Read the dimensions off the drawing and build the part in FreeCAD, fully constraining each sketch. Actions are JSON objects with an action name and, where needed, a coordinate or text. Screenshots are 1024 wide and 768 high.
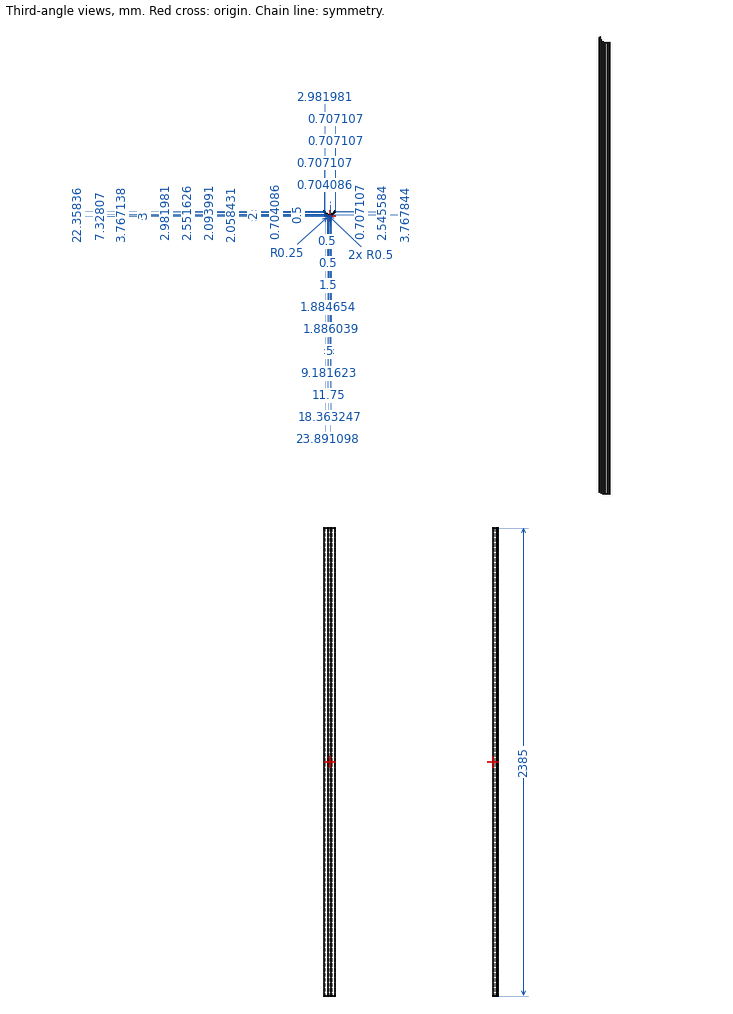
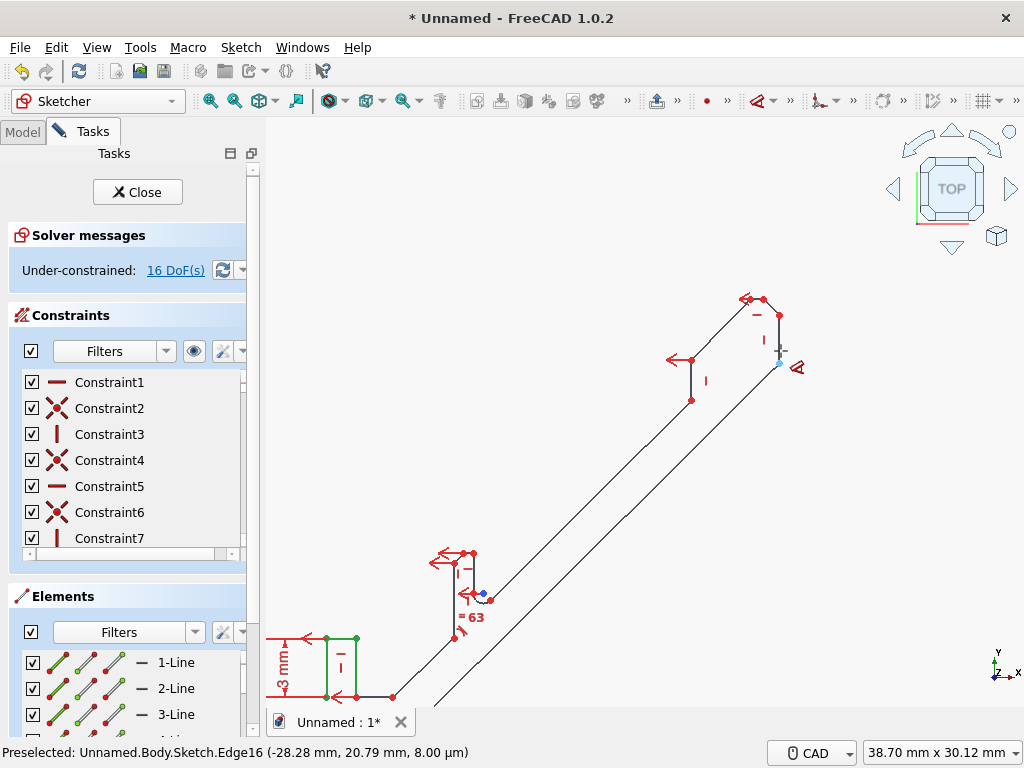
{"action": "left_click", "coordinate": [779, 349]}
{"action": "left_click", "coordinate": [813, 339]}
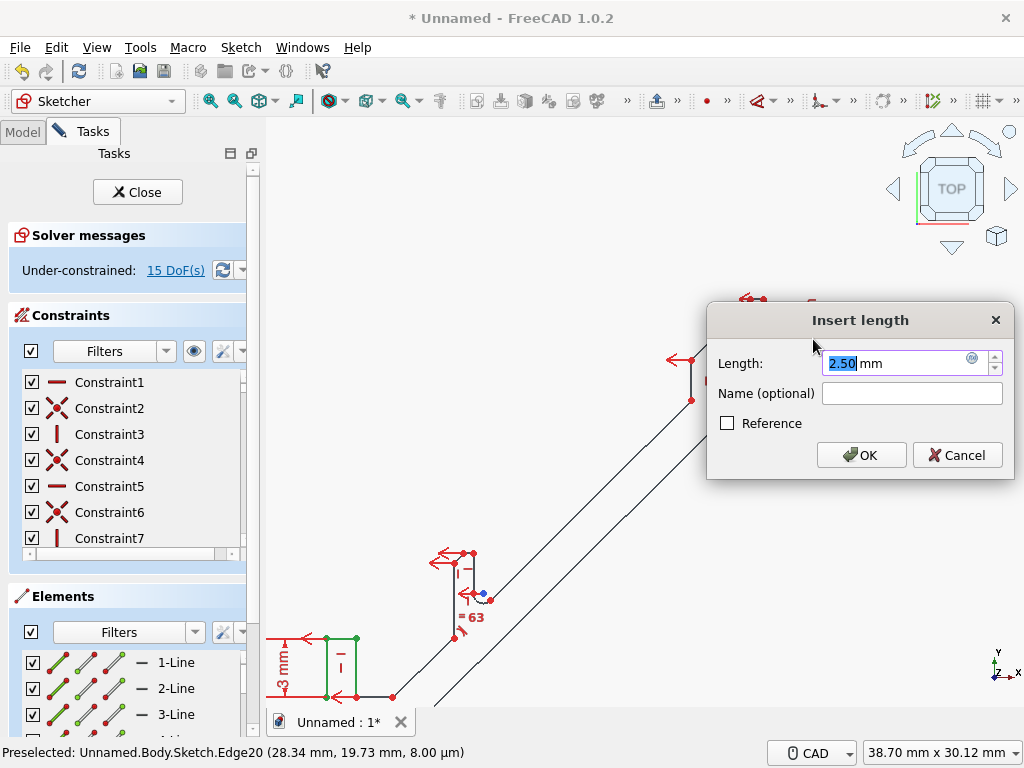
{"action": "type", "text": "2.545584"}
{"action": "key", "text": "Return"}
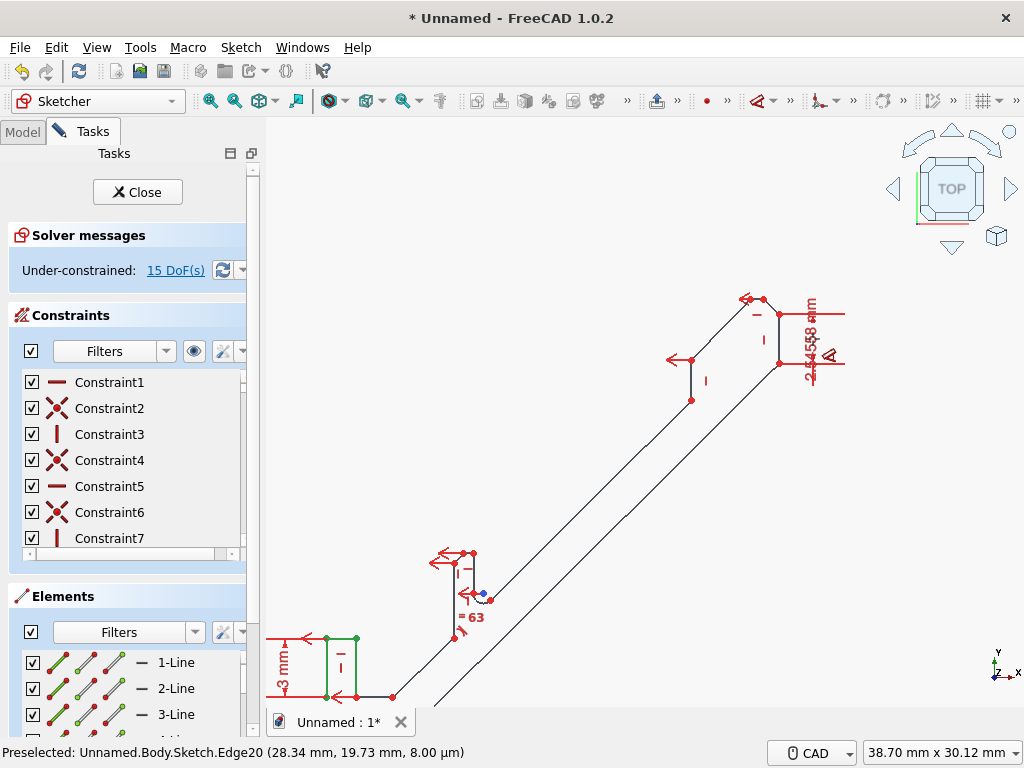
{"action": "scroll", "coordinate": [757, 299], "scroll_direction": "up", "scroll_amount": 6}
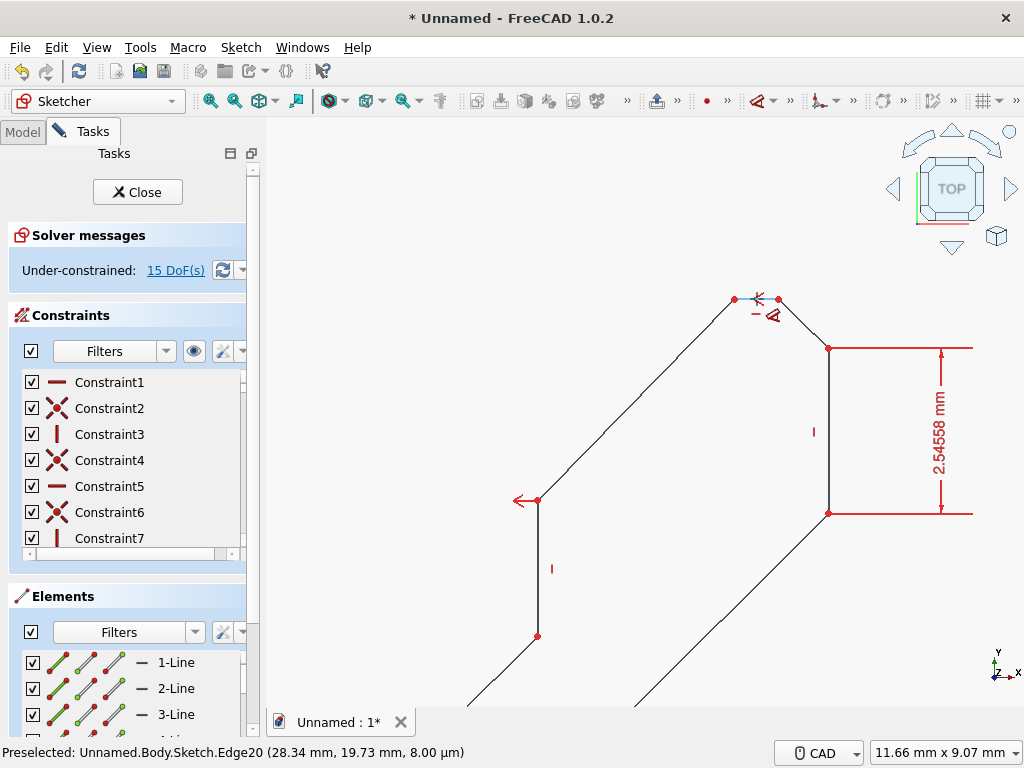
{"action": "left_click", "coordinate": [756, 299]}
{"action": "left_click", "coordinate": [756, 265]}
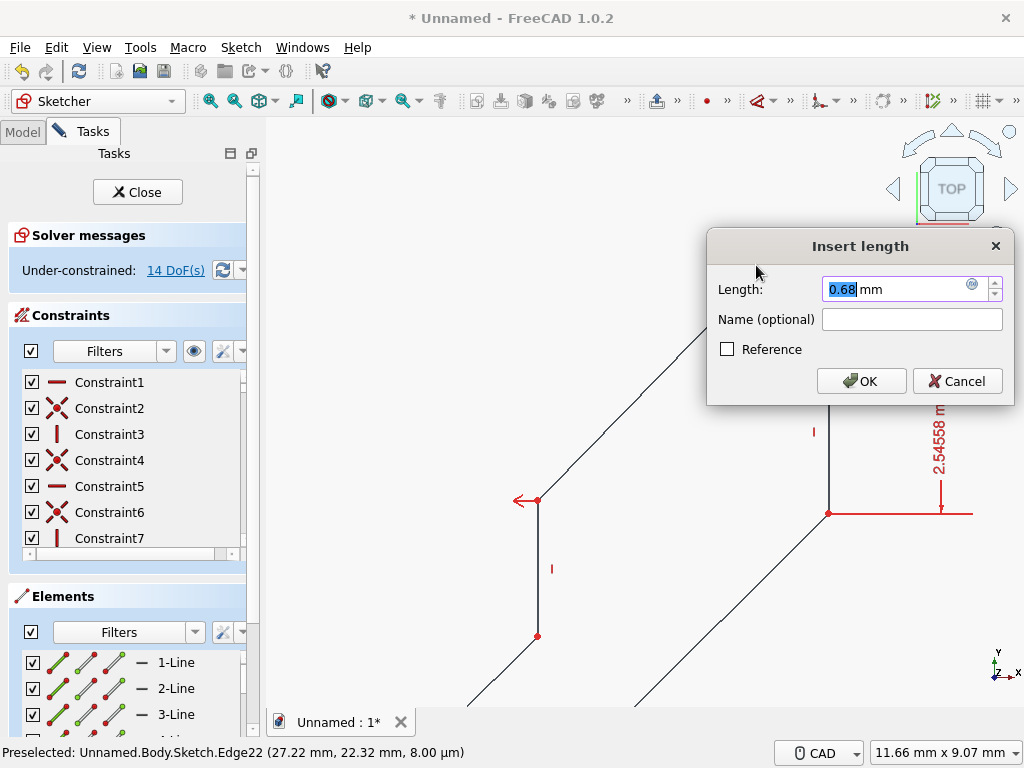
{"action": "type", "text": "0.707107"}
{"action": "key", "text": "Return"}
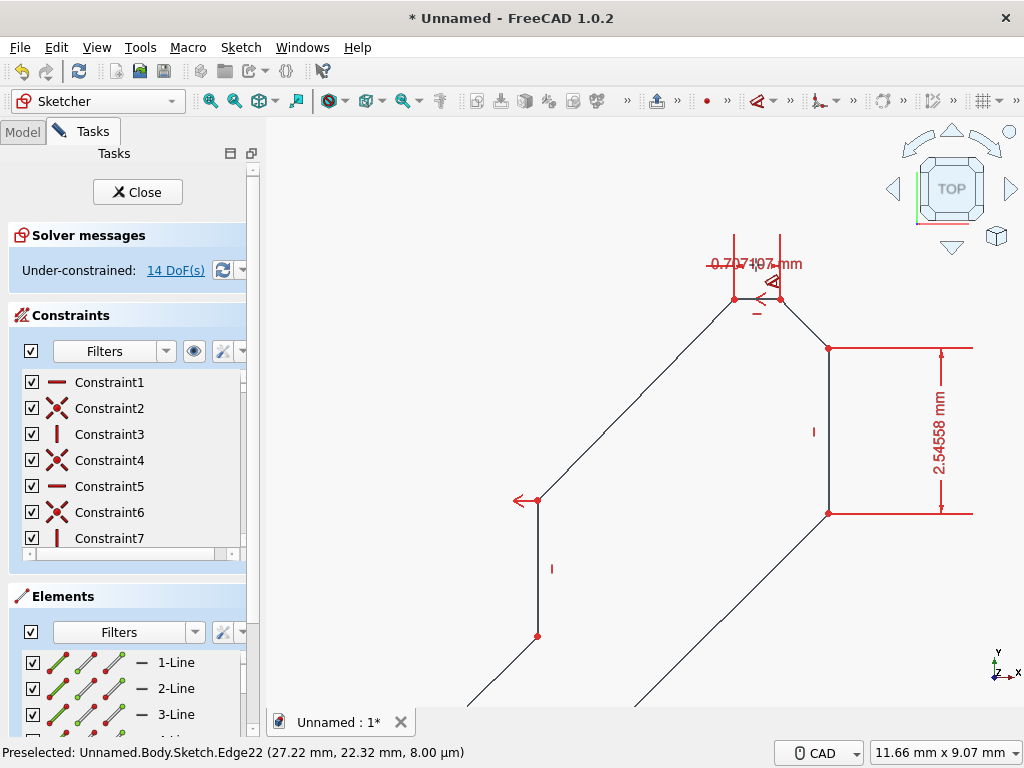
{"action": "scroll", "coordinate": [775, 336], "scroll_direction": "down", "scroll_amount": 11}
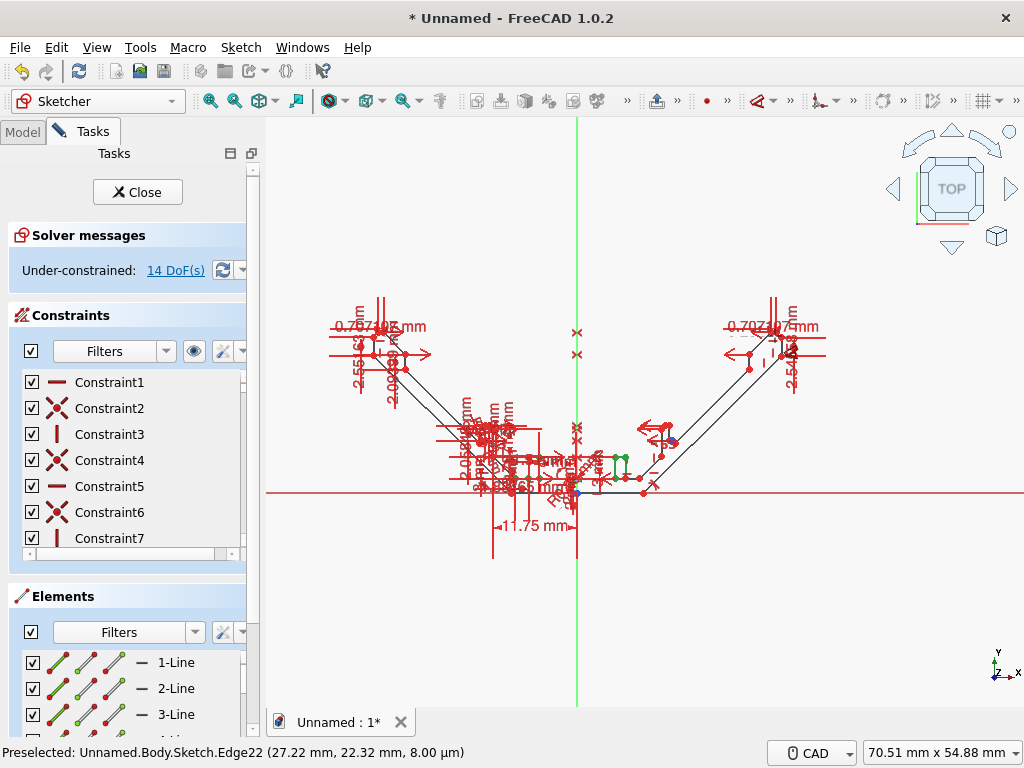
{"action": "scroll", "coordinate": [749, 359], "scroll_direction": "up", "scroll_amount": 6}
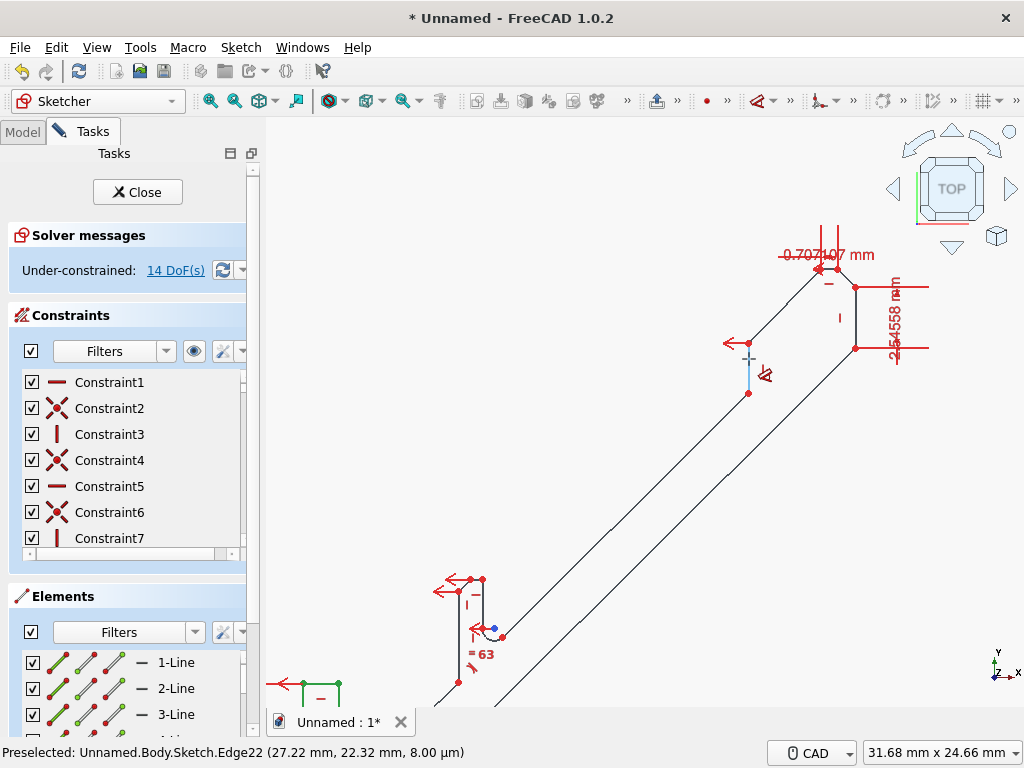
{"action": "left_click", "coordinate": [749, 358]}
{"action": "left_click", "coordinate": [783, 368]}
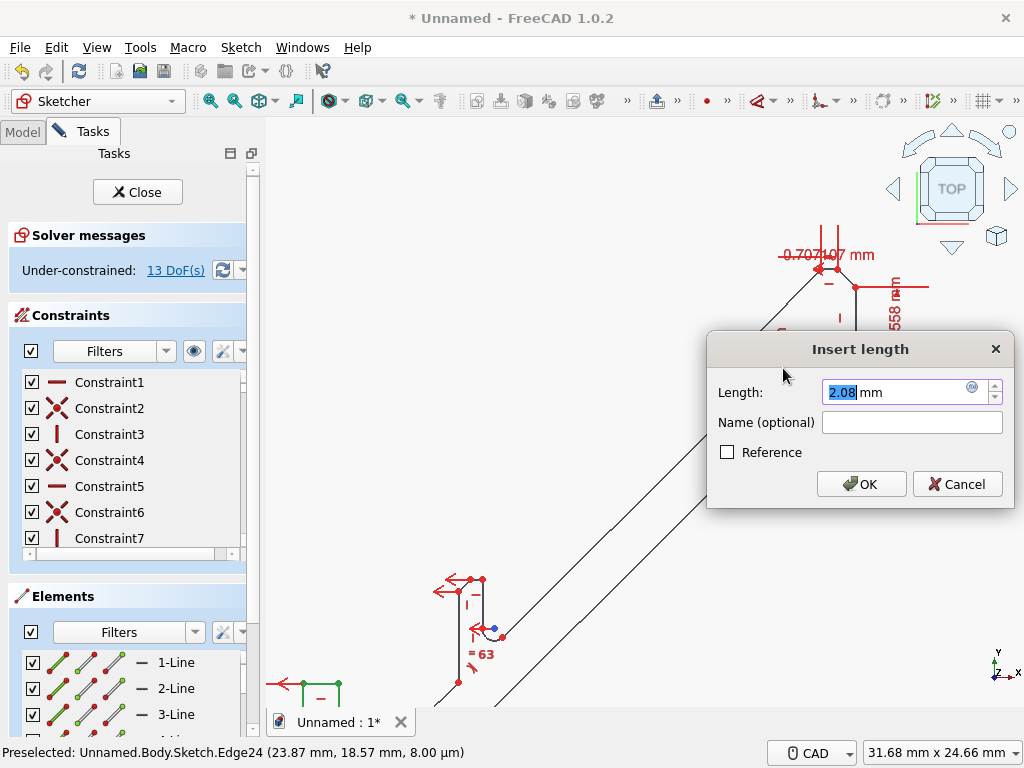
{"action": "type", "text": "2.093991"}
{"action": "key", "text": "Return"}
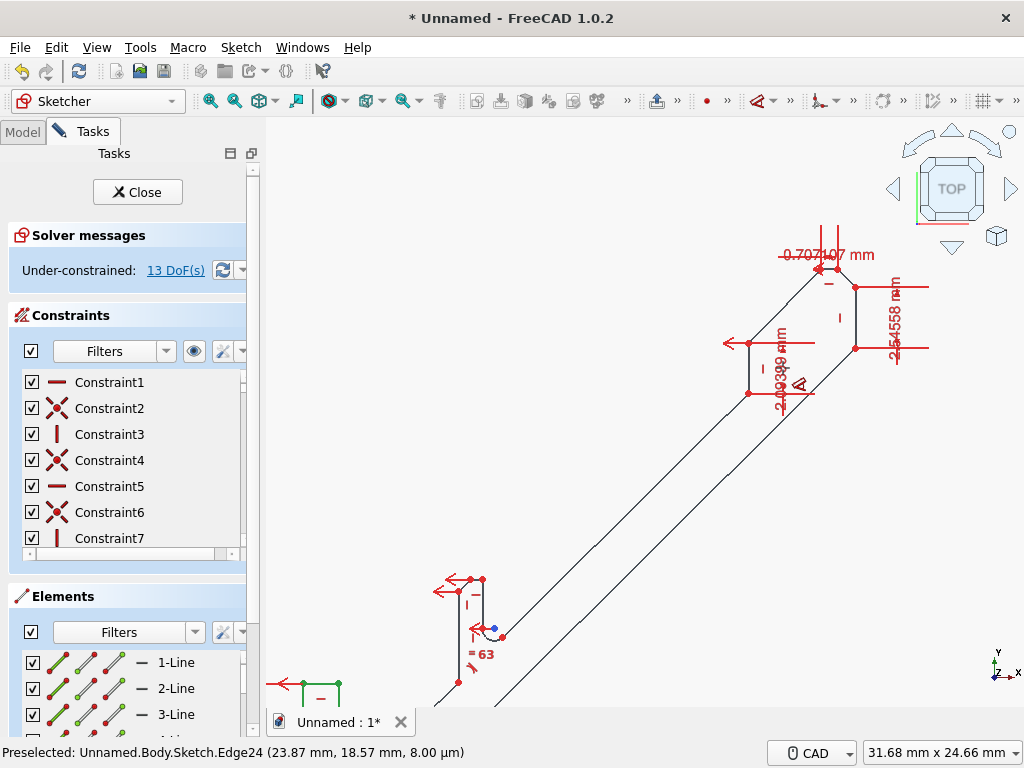
{"action": "left_click", "coordinate": [459, 619]}
{"action": "left_click", "coordinate": [493, 655]}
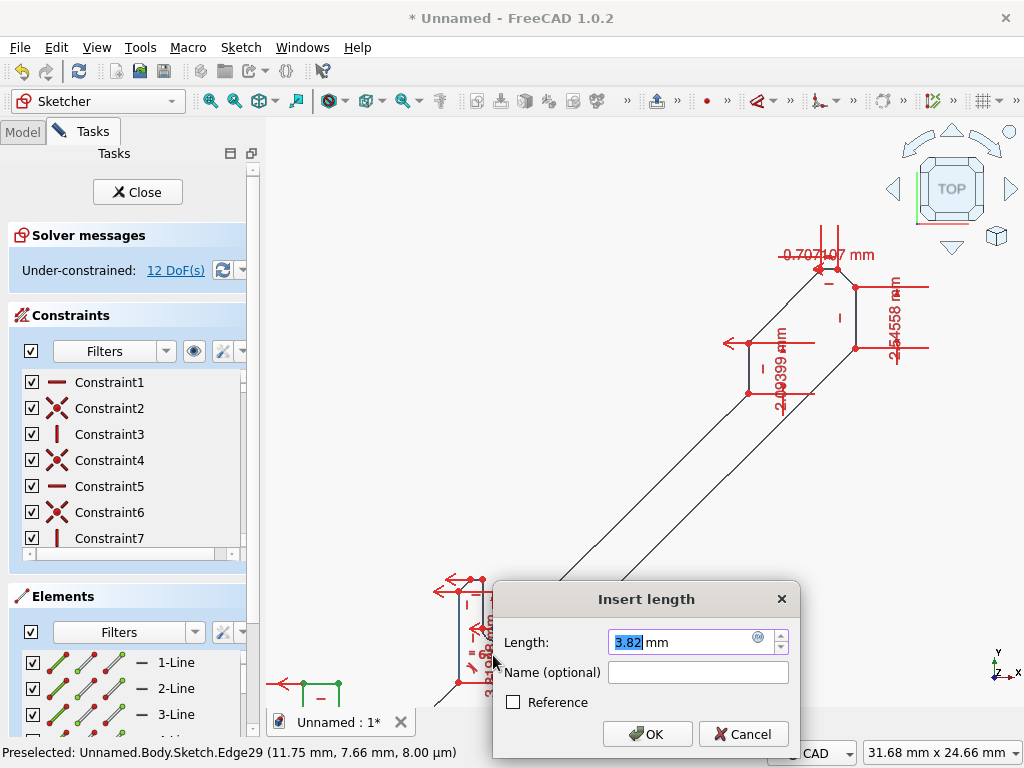
{"action": "type", "text": "3.767844"}
{"action": "key", "text": "Return"}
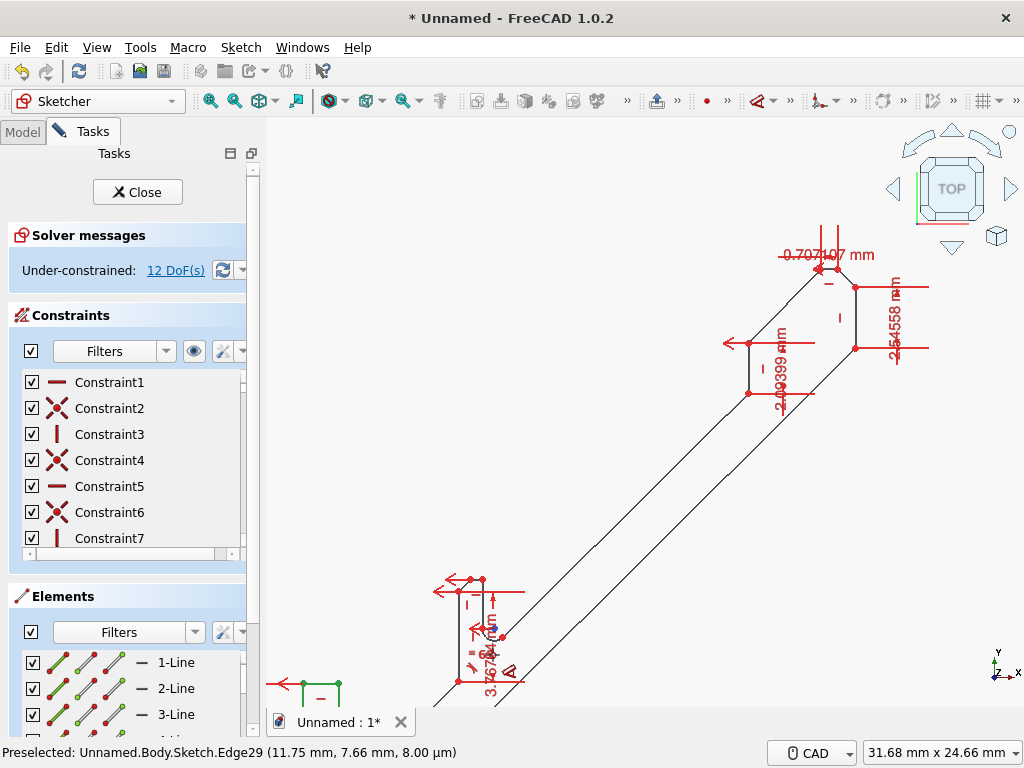
{"action": "scroll", "coordinate": [748, 359], "scroll_direction": "down", "scroll_amount": 6}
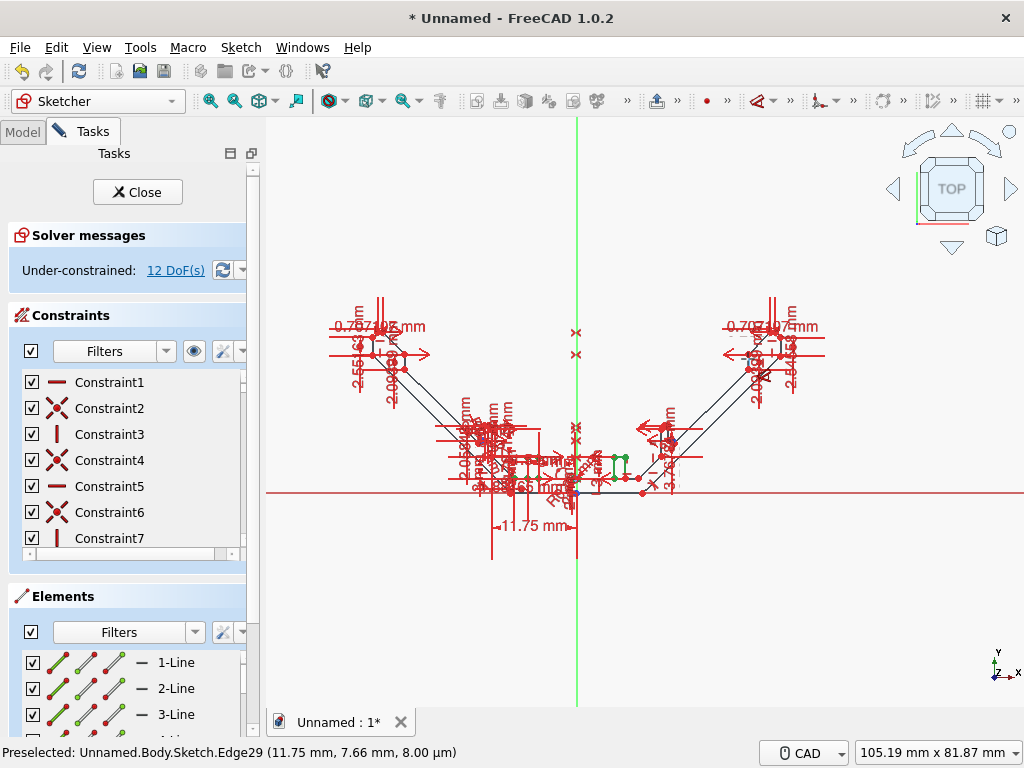
{"action": "scroll", "coordinate": [635, 479], "scroll_direction": "up", "scroll_amount": 7}